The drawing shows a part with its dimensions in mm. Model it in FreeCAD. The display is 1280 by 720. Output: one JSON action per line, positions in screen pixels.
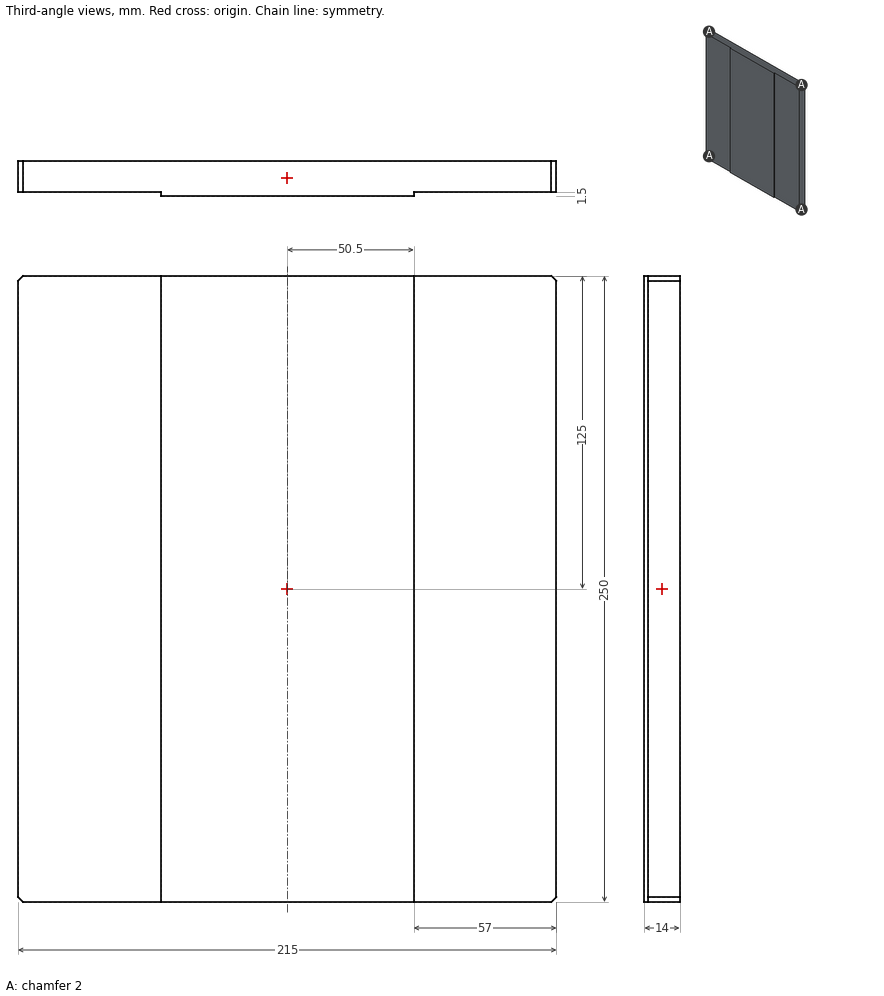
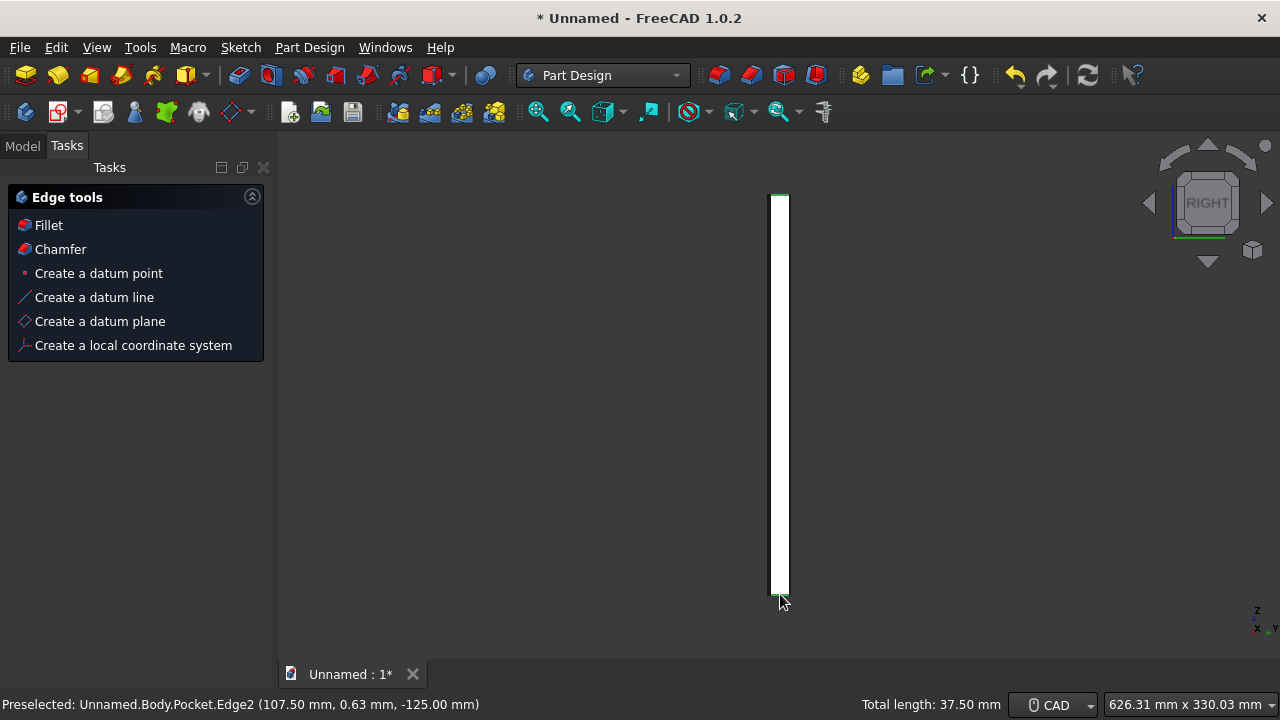
{"action": "key", "text": "5"}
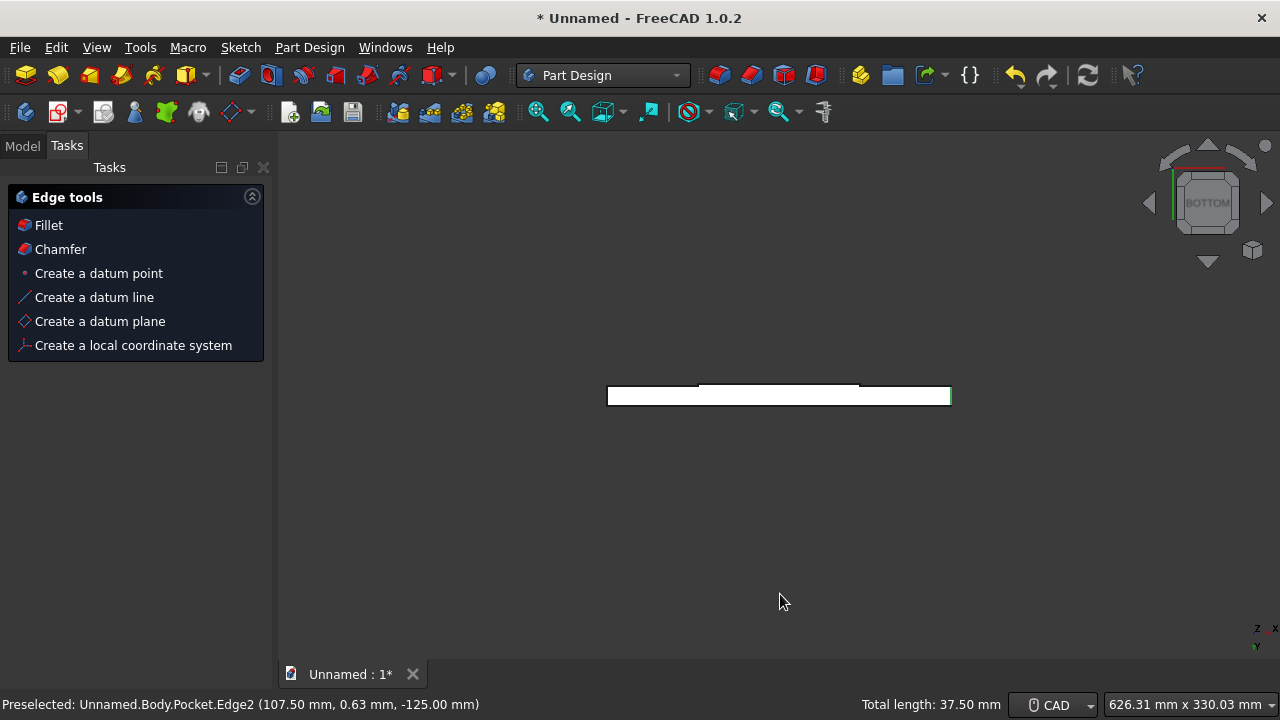
{"action": "key", "text": "v f"}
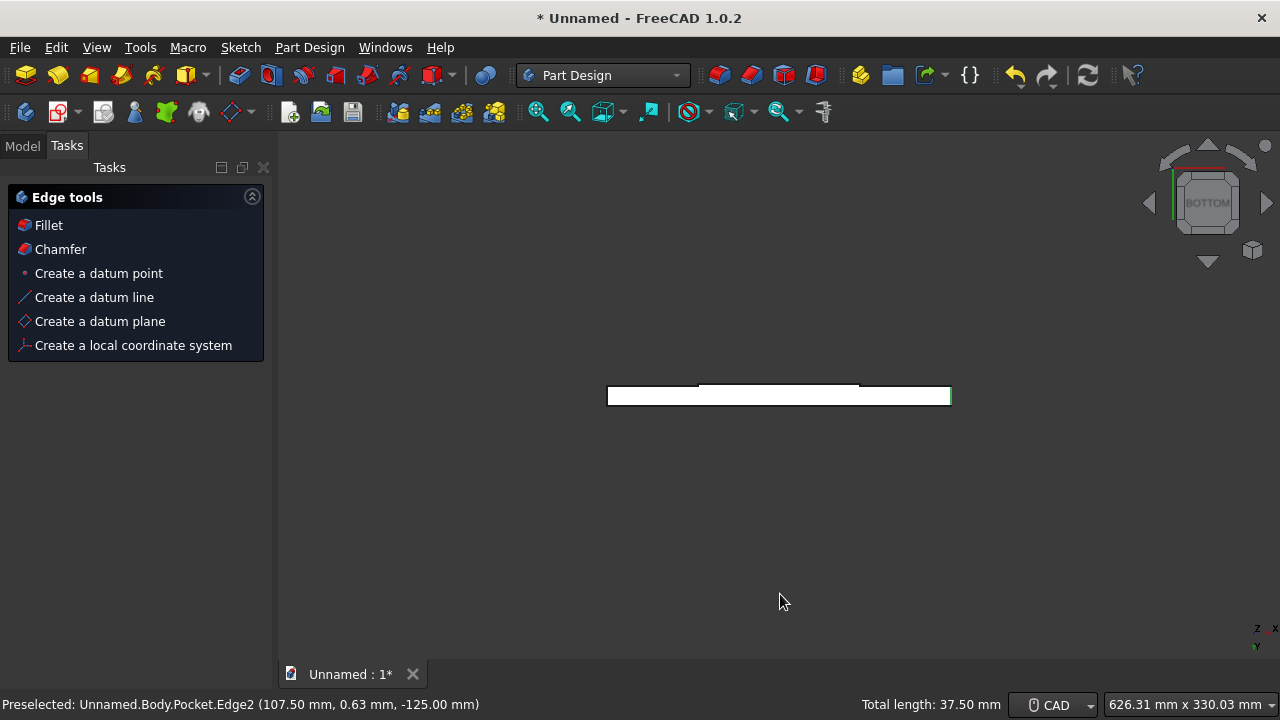
{"action": "left_click", "coordinate": [607, 395], "text": "ctrl"}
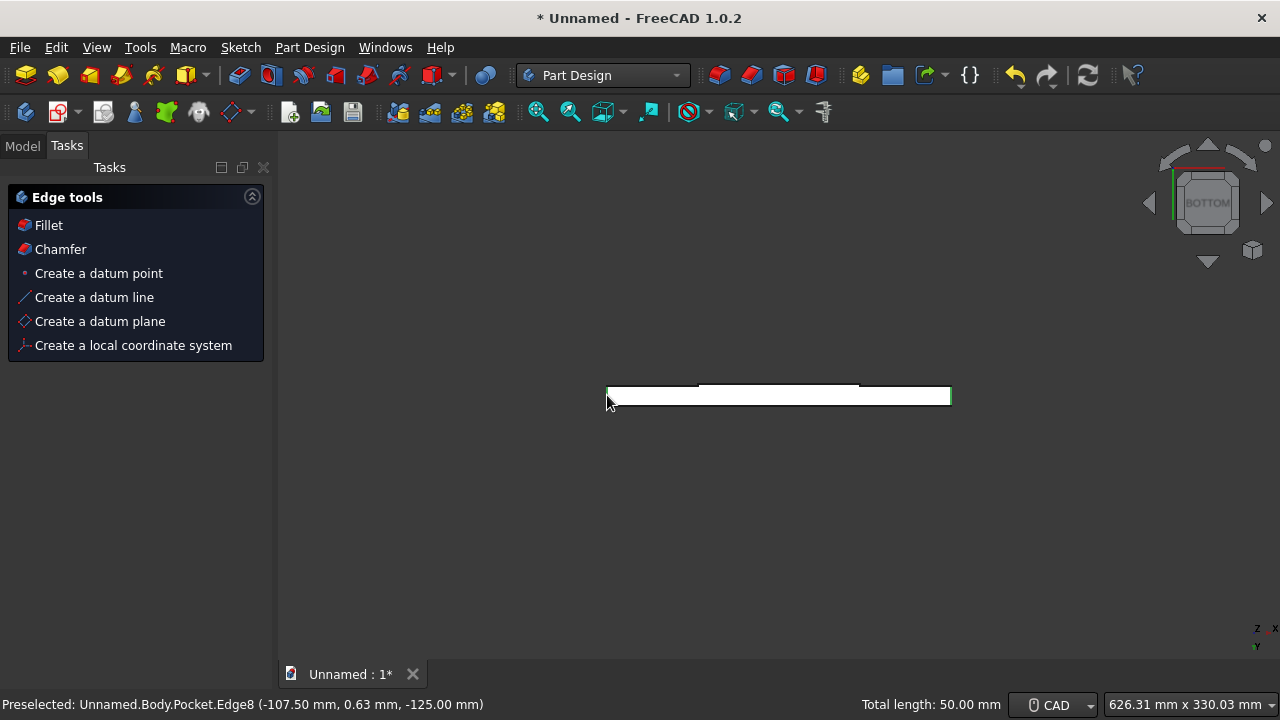
{"action": "left_click", "coordinate": [752, 76]}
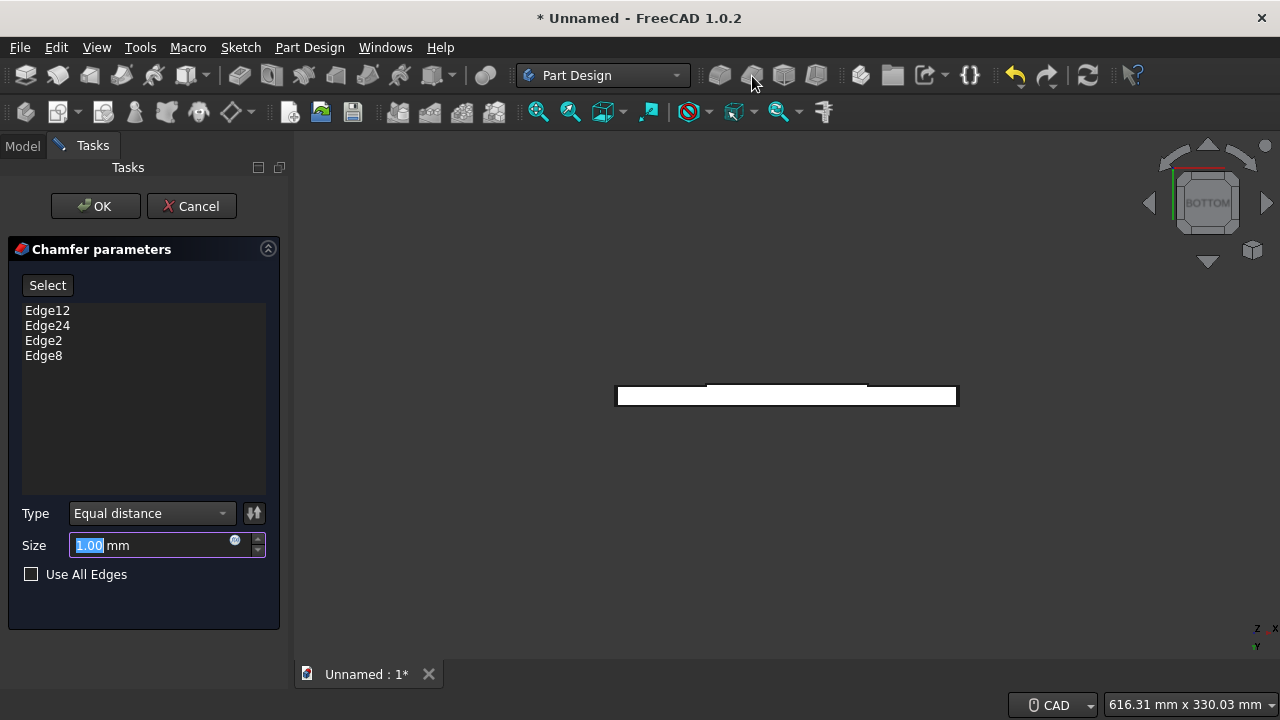
{"action": "type", "text": "2"}
{"action": "key", "text": "Tab"}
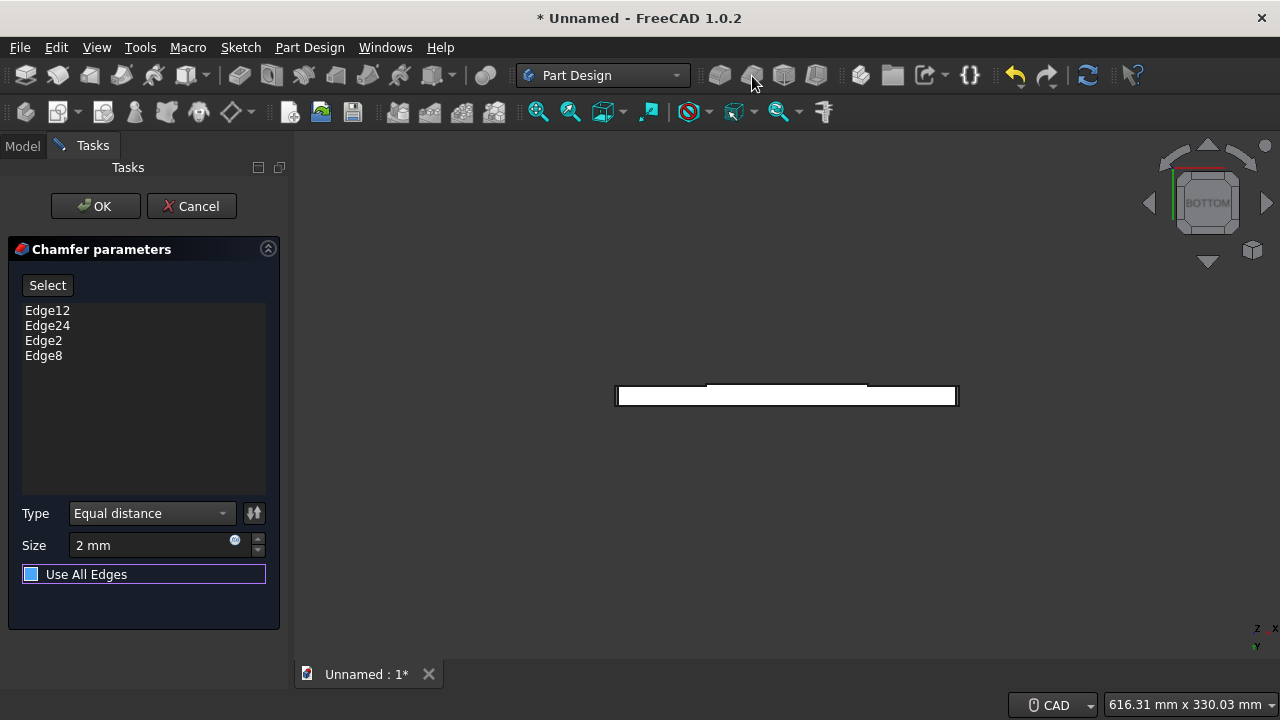
{"action": "left_click", "coordinate": [96, 206]}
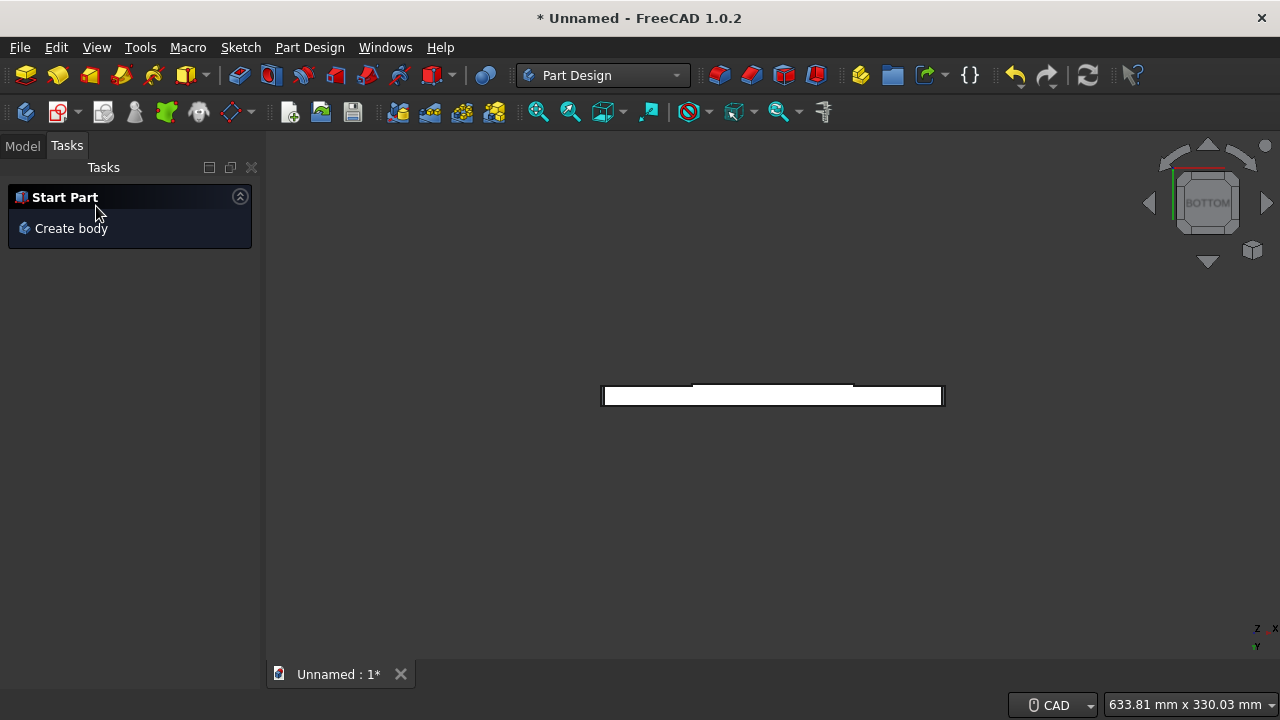
{"action": "key", "text": "0"}